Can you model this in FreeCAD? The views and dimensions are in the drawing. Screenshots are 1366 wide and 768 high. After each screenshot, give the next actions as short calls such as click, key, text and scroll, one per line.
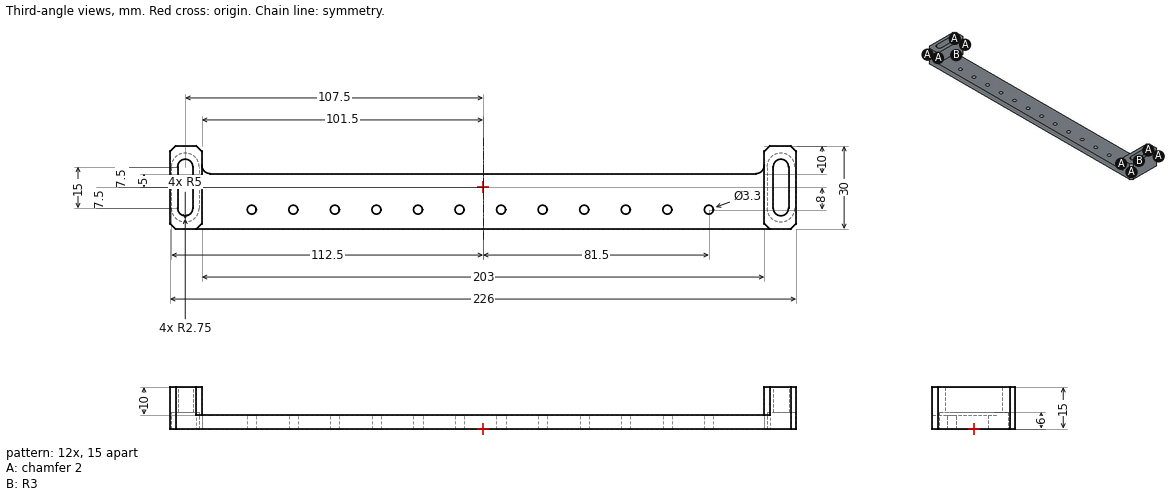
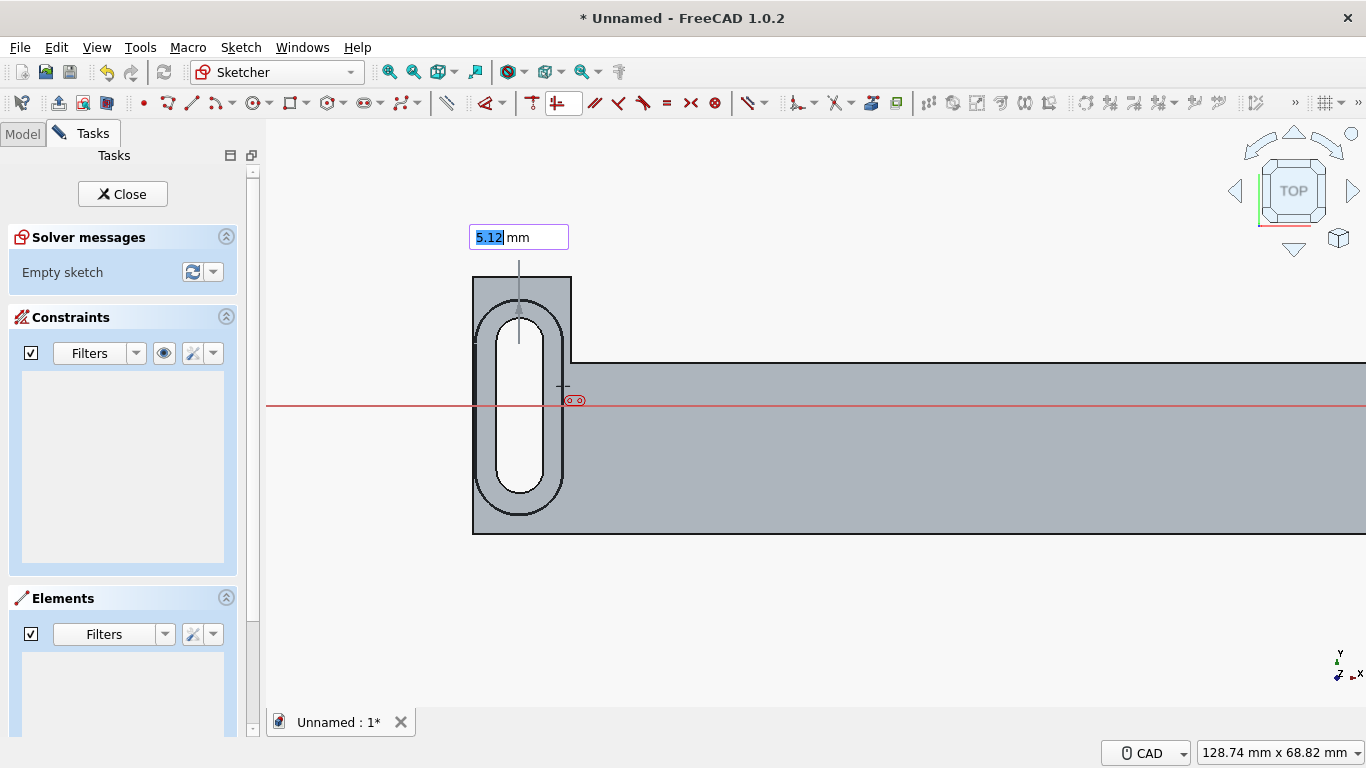
click(563, 386)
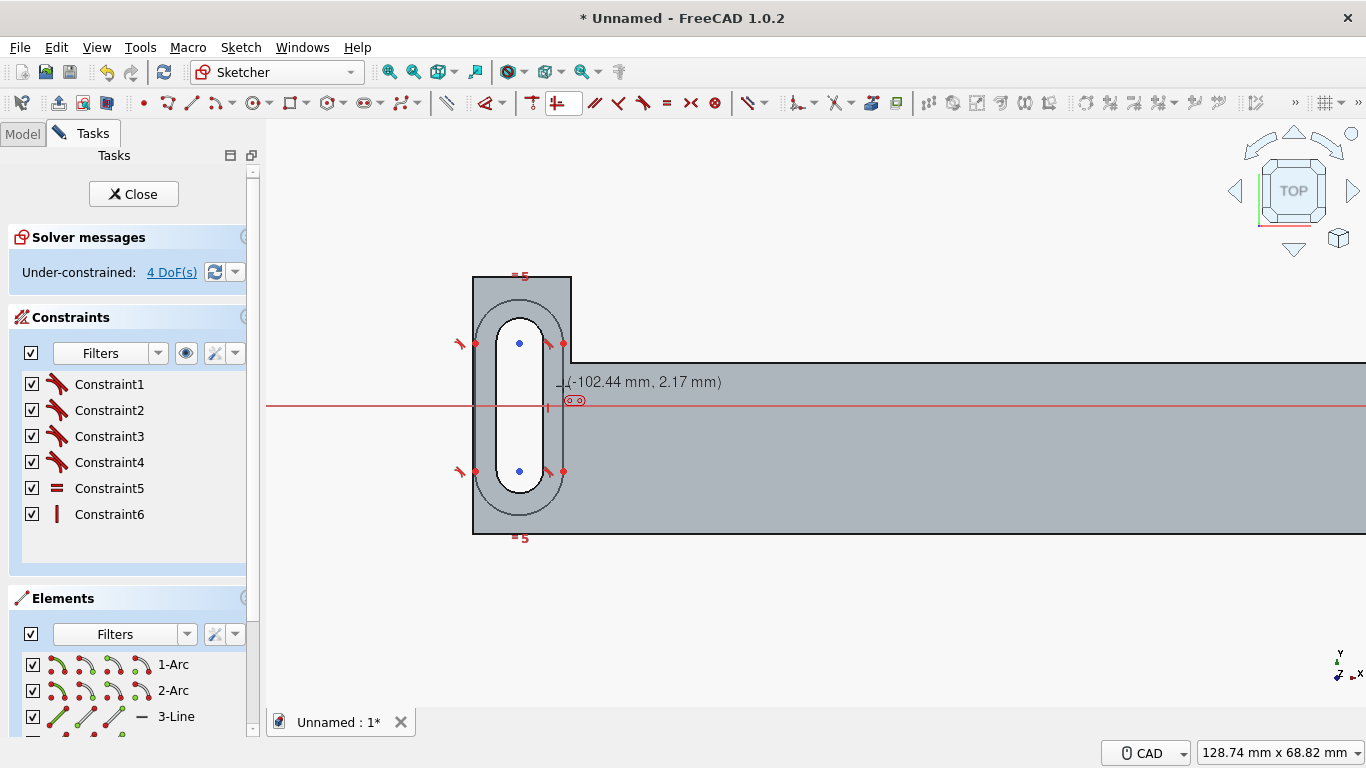
scroll(345, 417, down, 5)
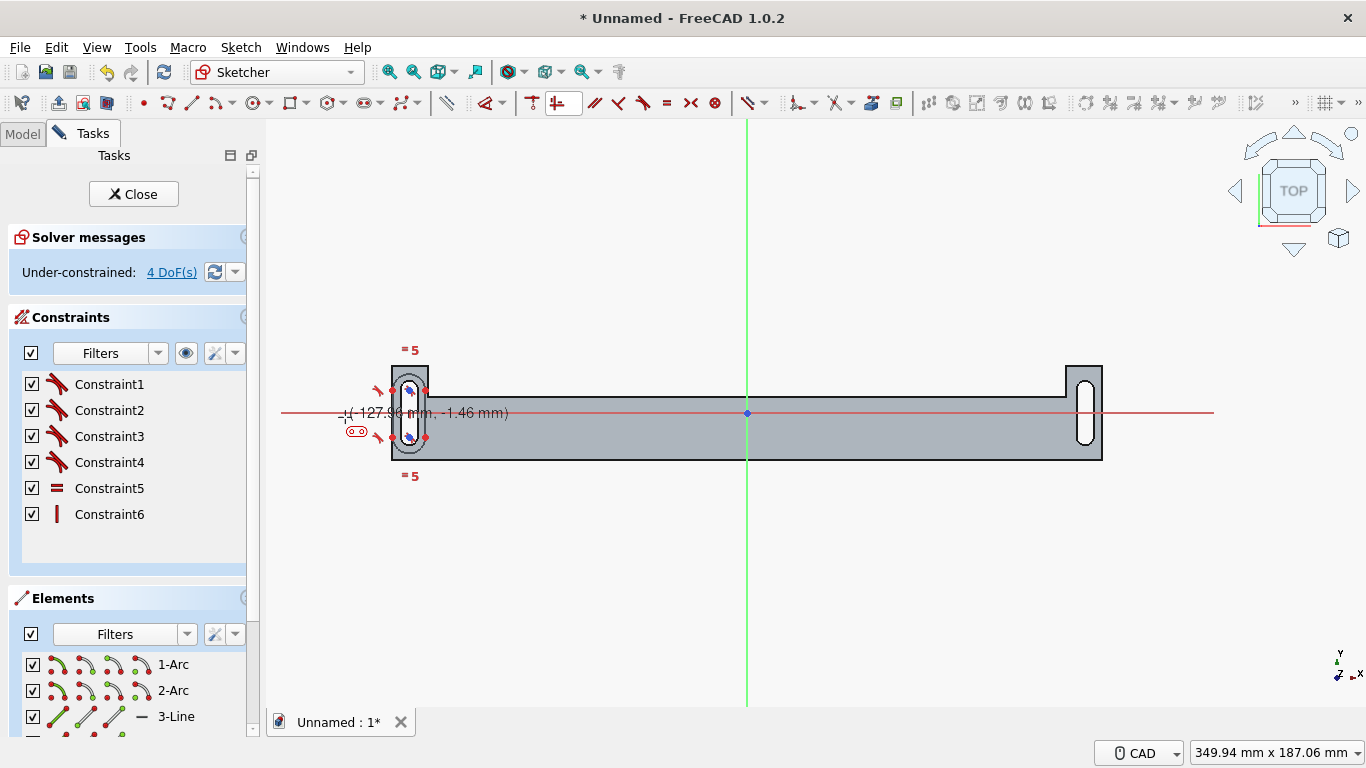
scroll(1085, 437, up, 2)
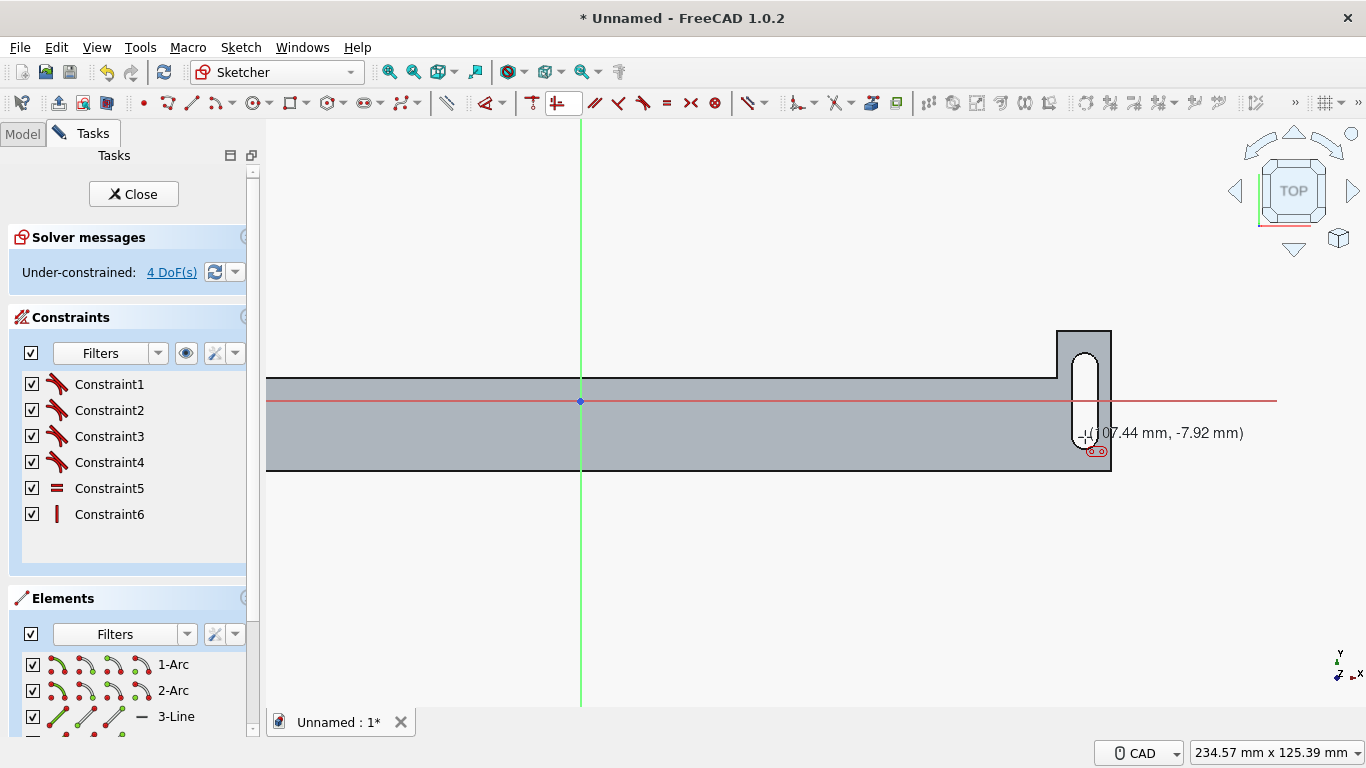
click(1085, 436)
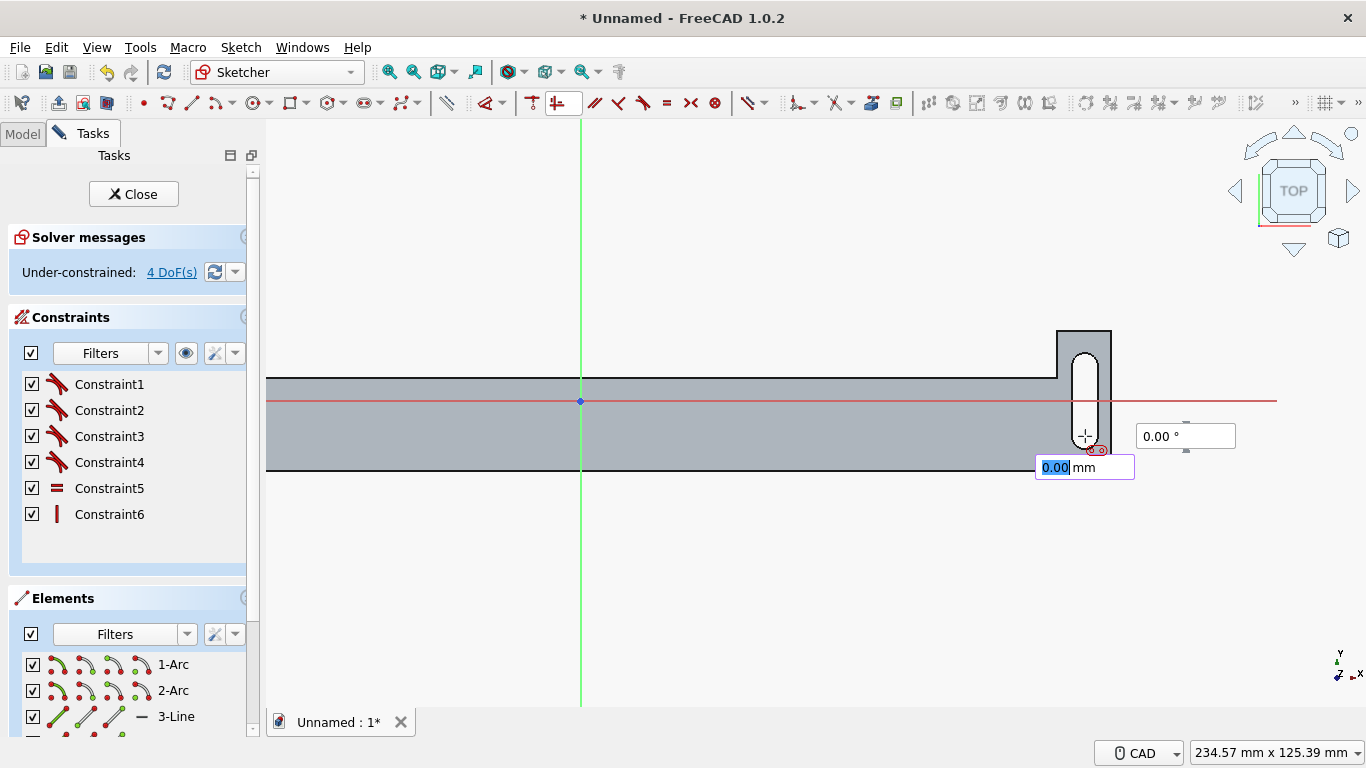
click(1085, 366)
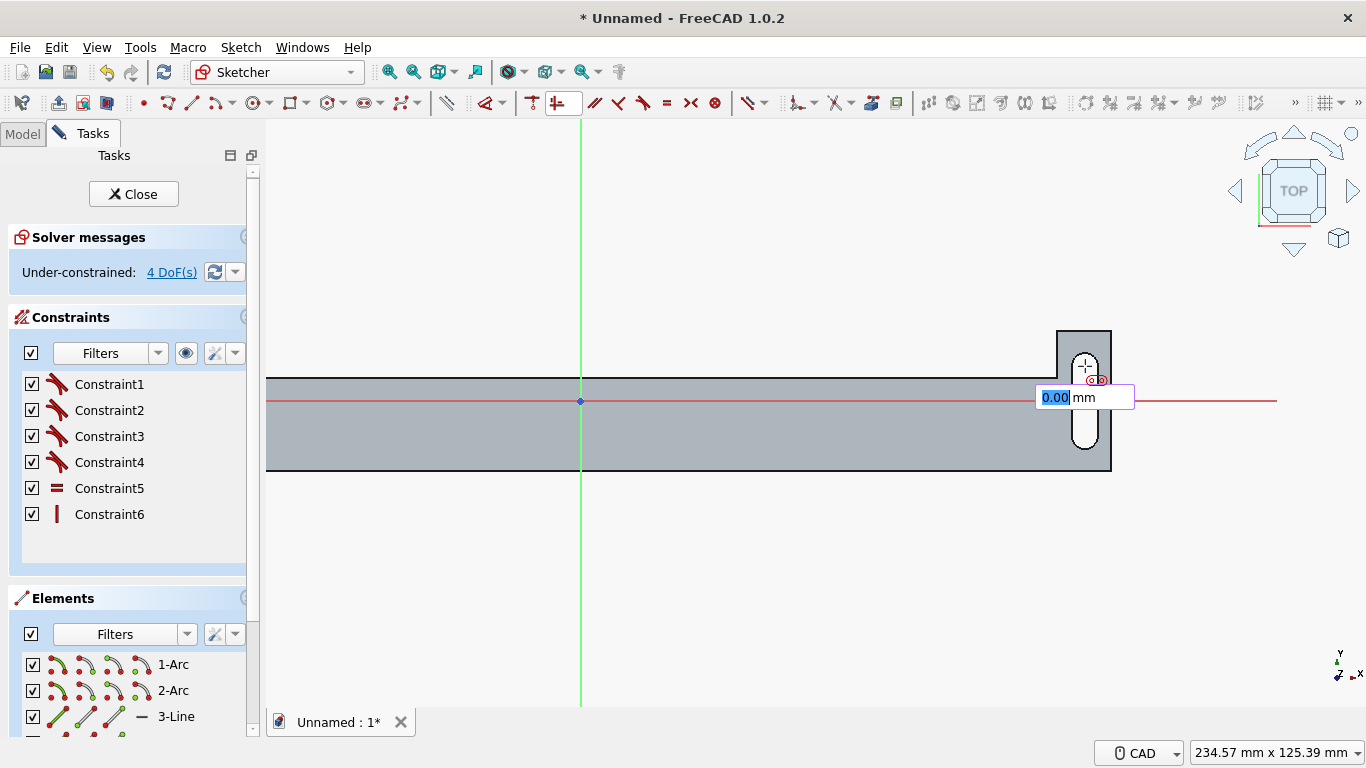
scroll(1108, 391, up, 3)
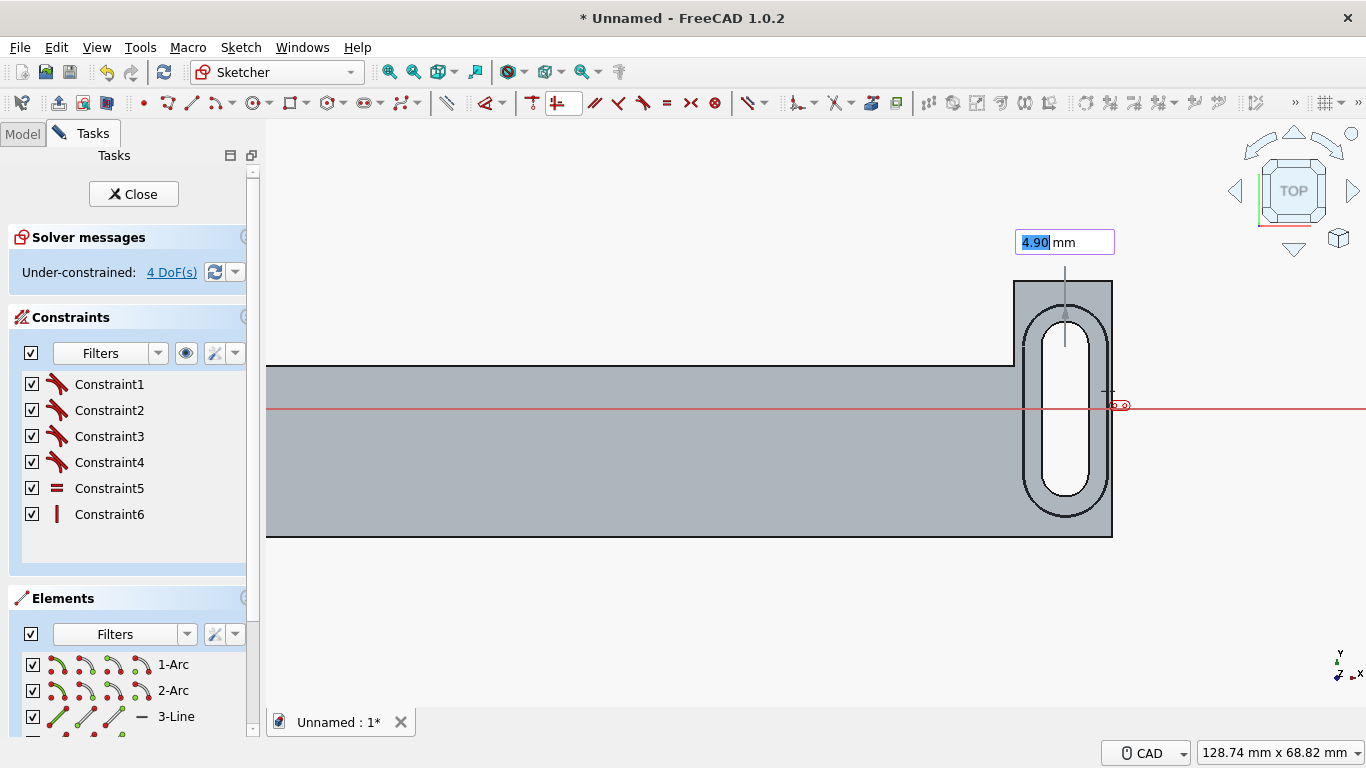
click(1108, 390)
key(Escape)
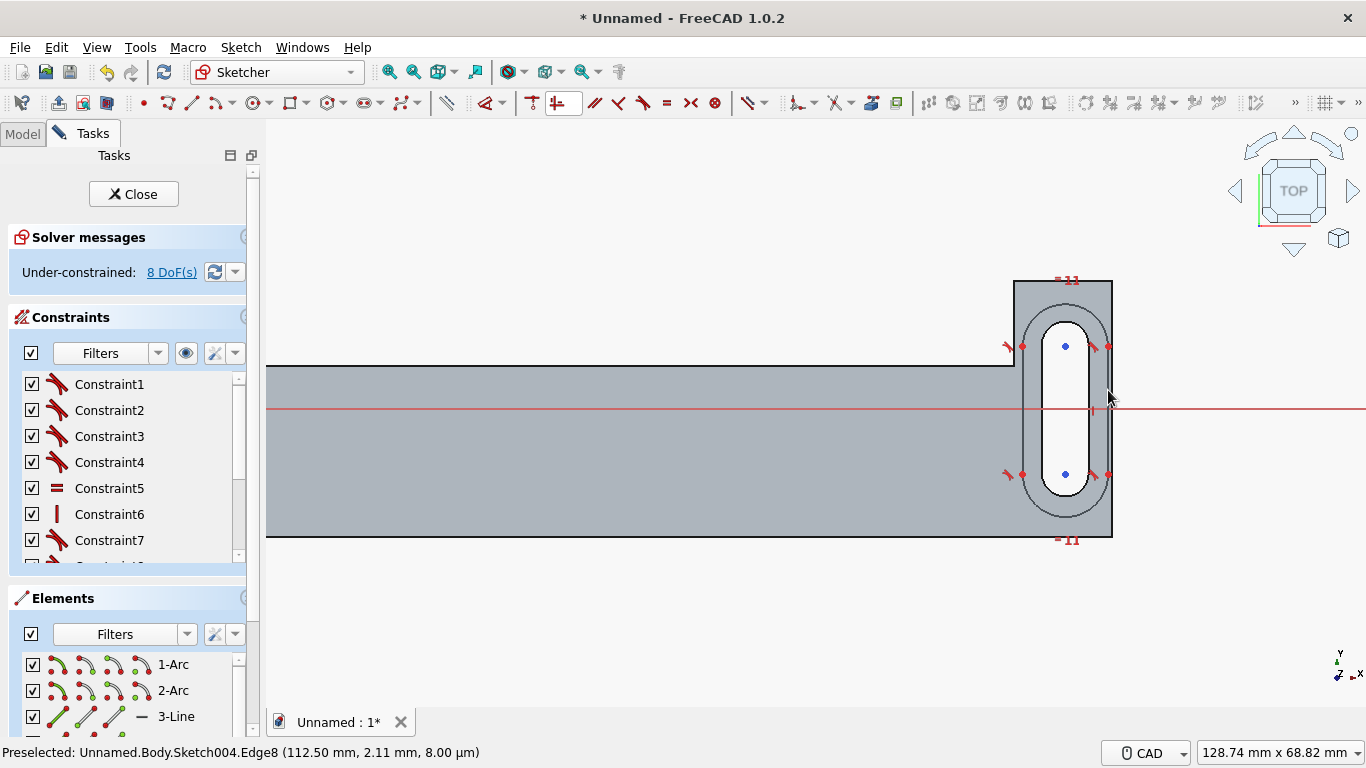
scroll(1097, 415, down, 5)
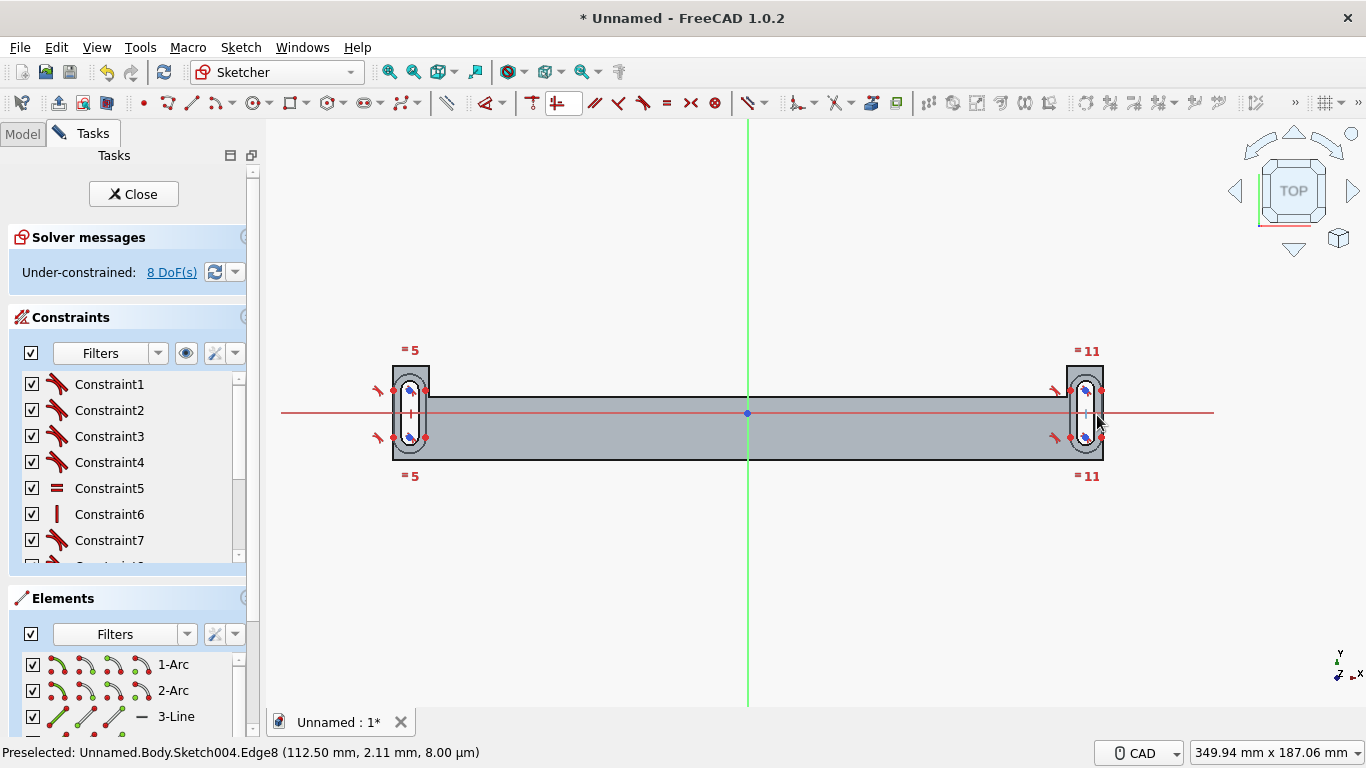
click(400, 450)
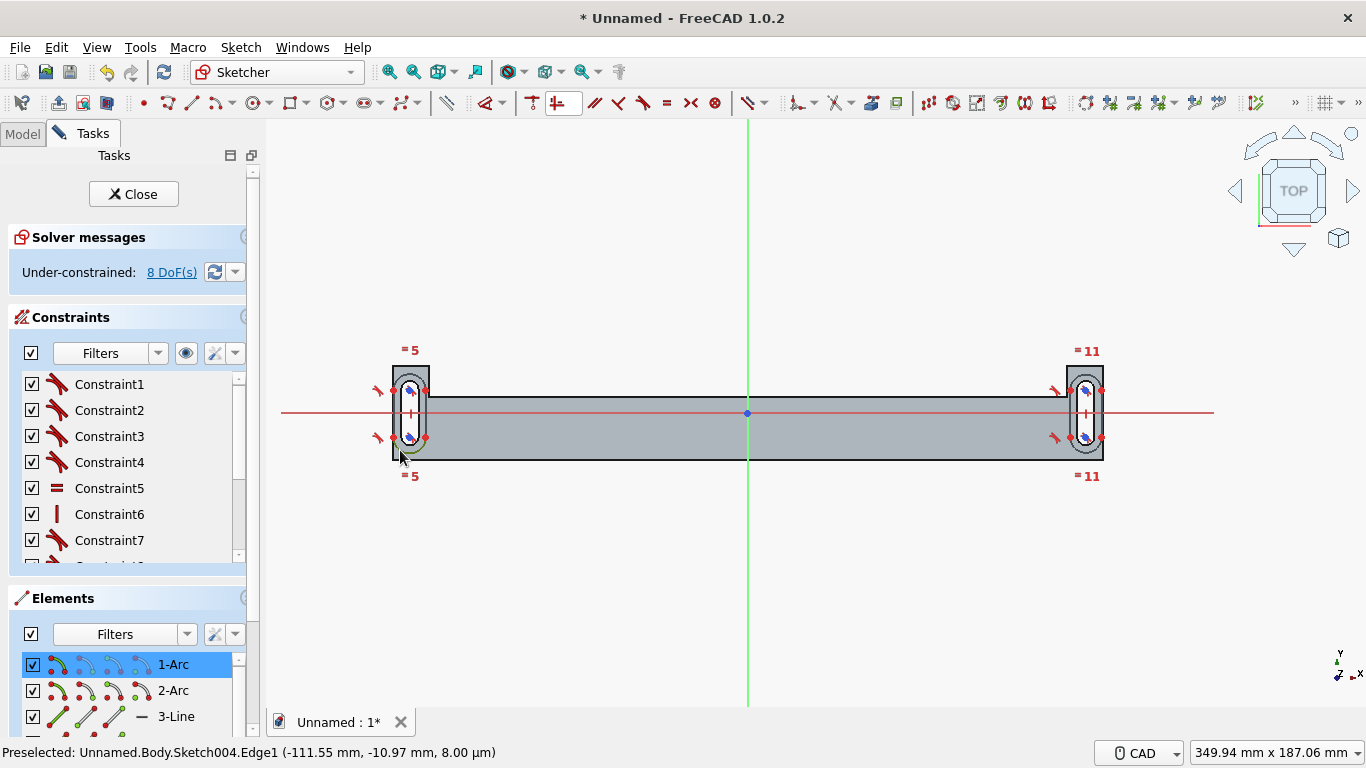
click(1077, 450)